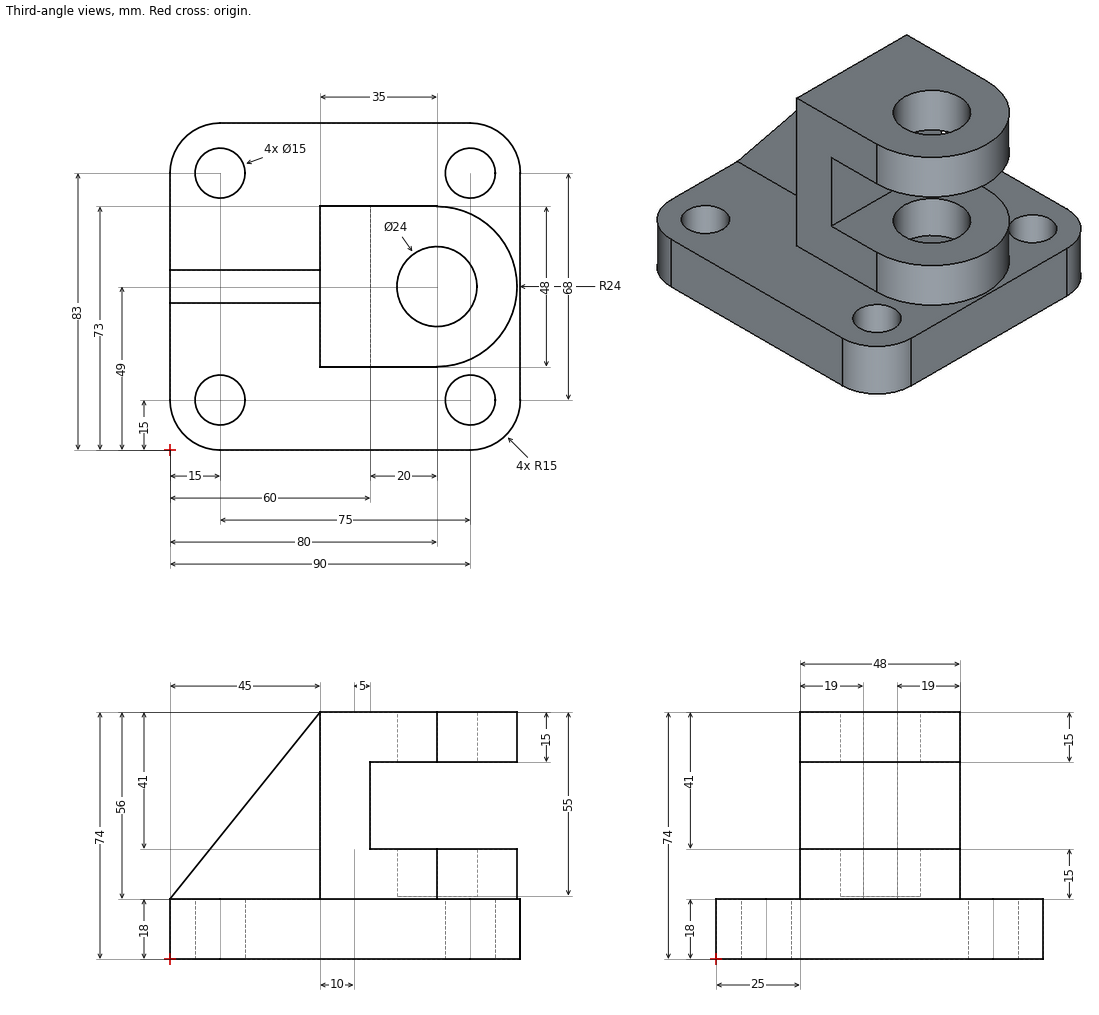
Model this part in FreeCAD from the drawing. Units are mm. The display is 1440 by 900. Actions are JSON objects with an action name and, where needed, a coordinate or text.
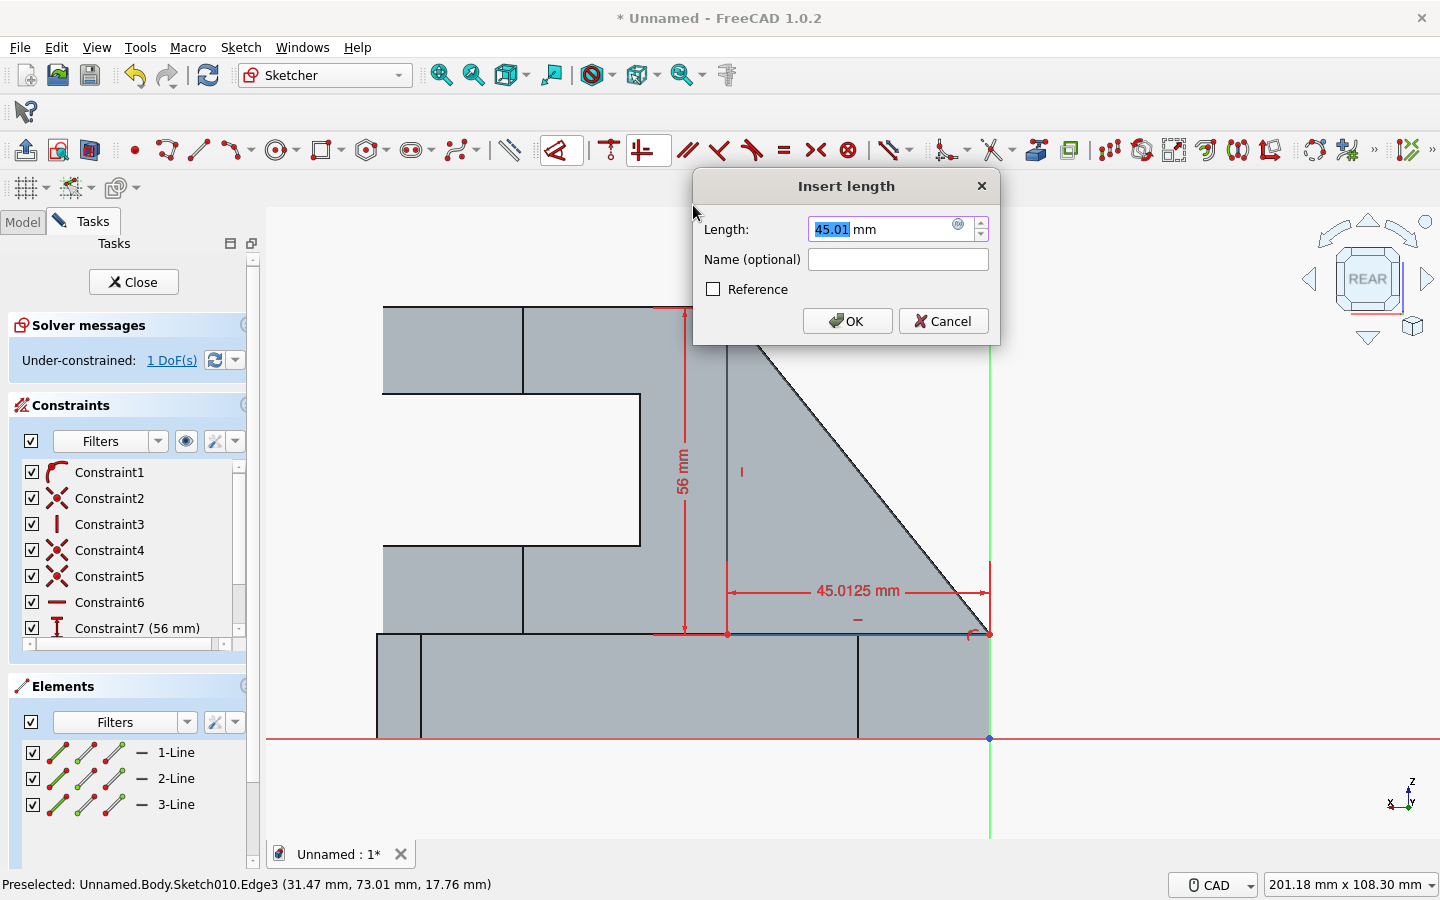
{"action": "type", "text": "45"}
{"action": "key", "text": "Return"}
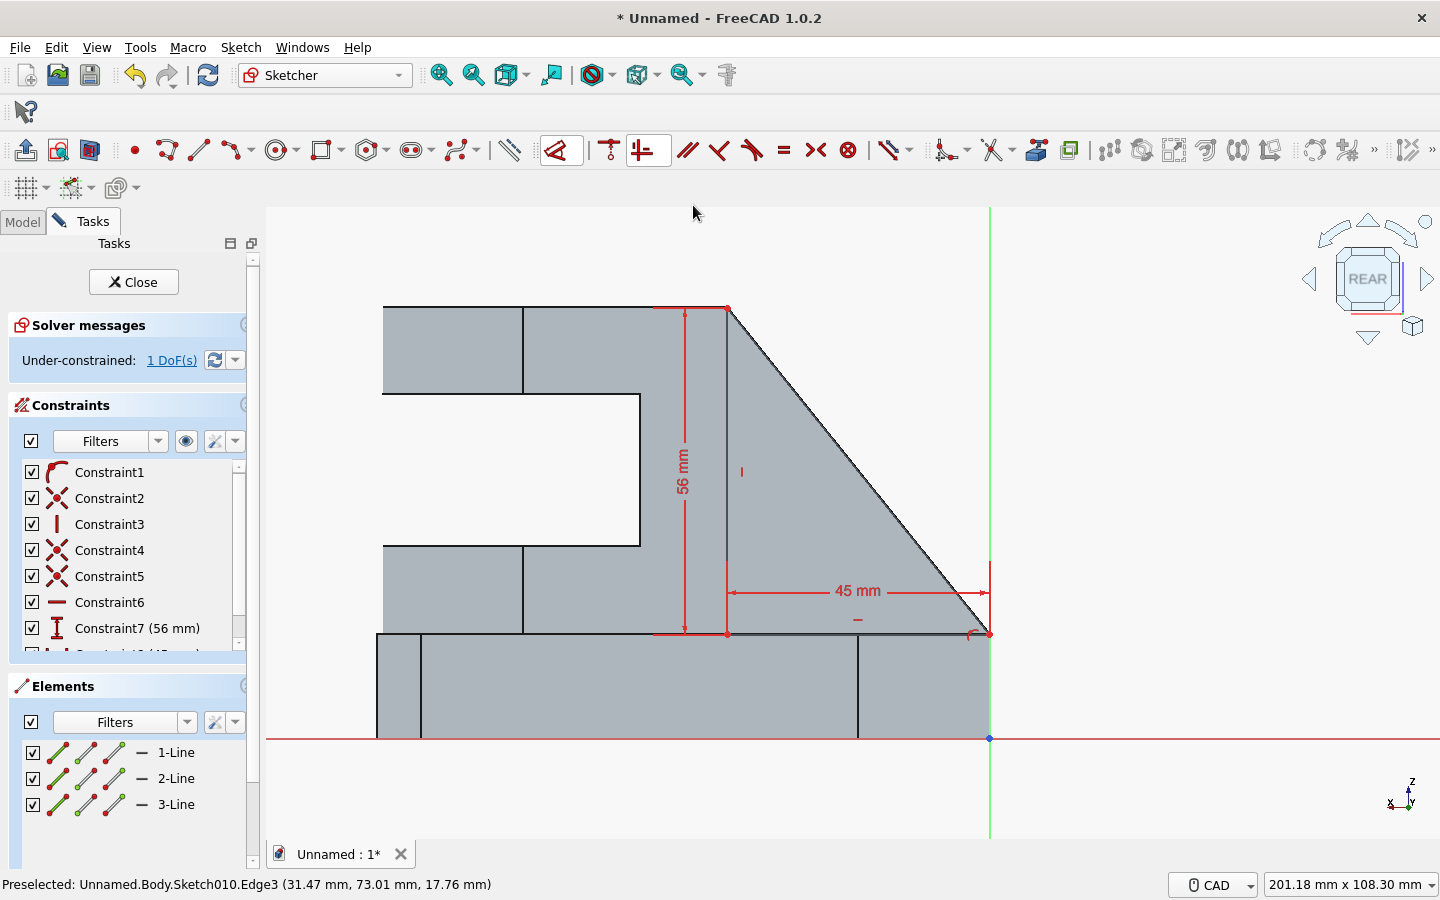
{"action": "left_click", "coordinate": [990, 635]}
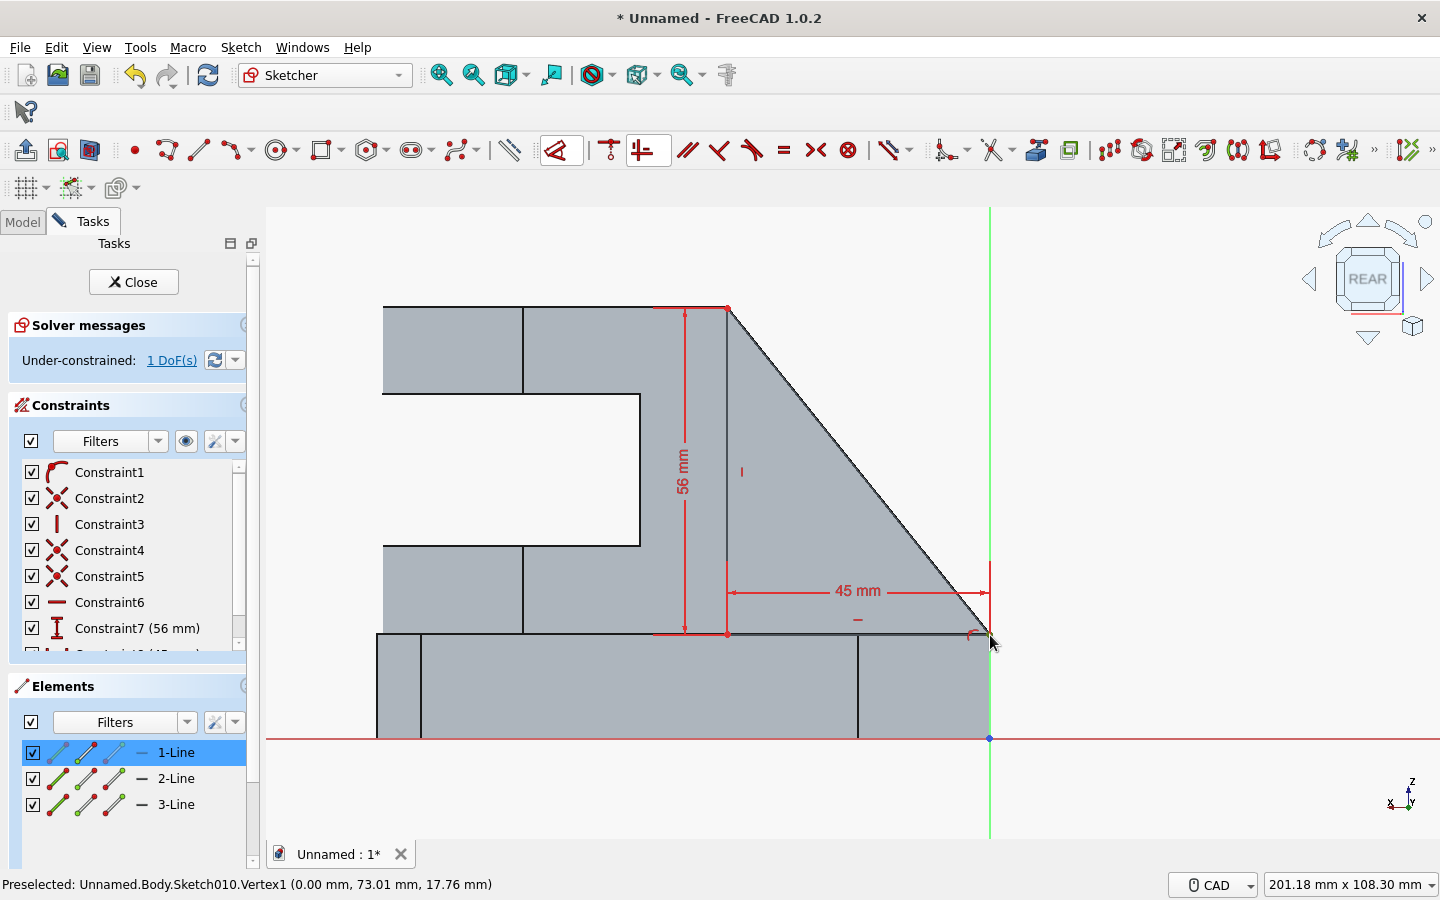
{"action": "left_click", "coordinate": [578, 150]}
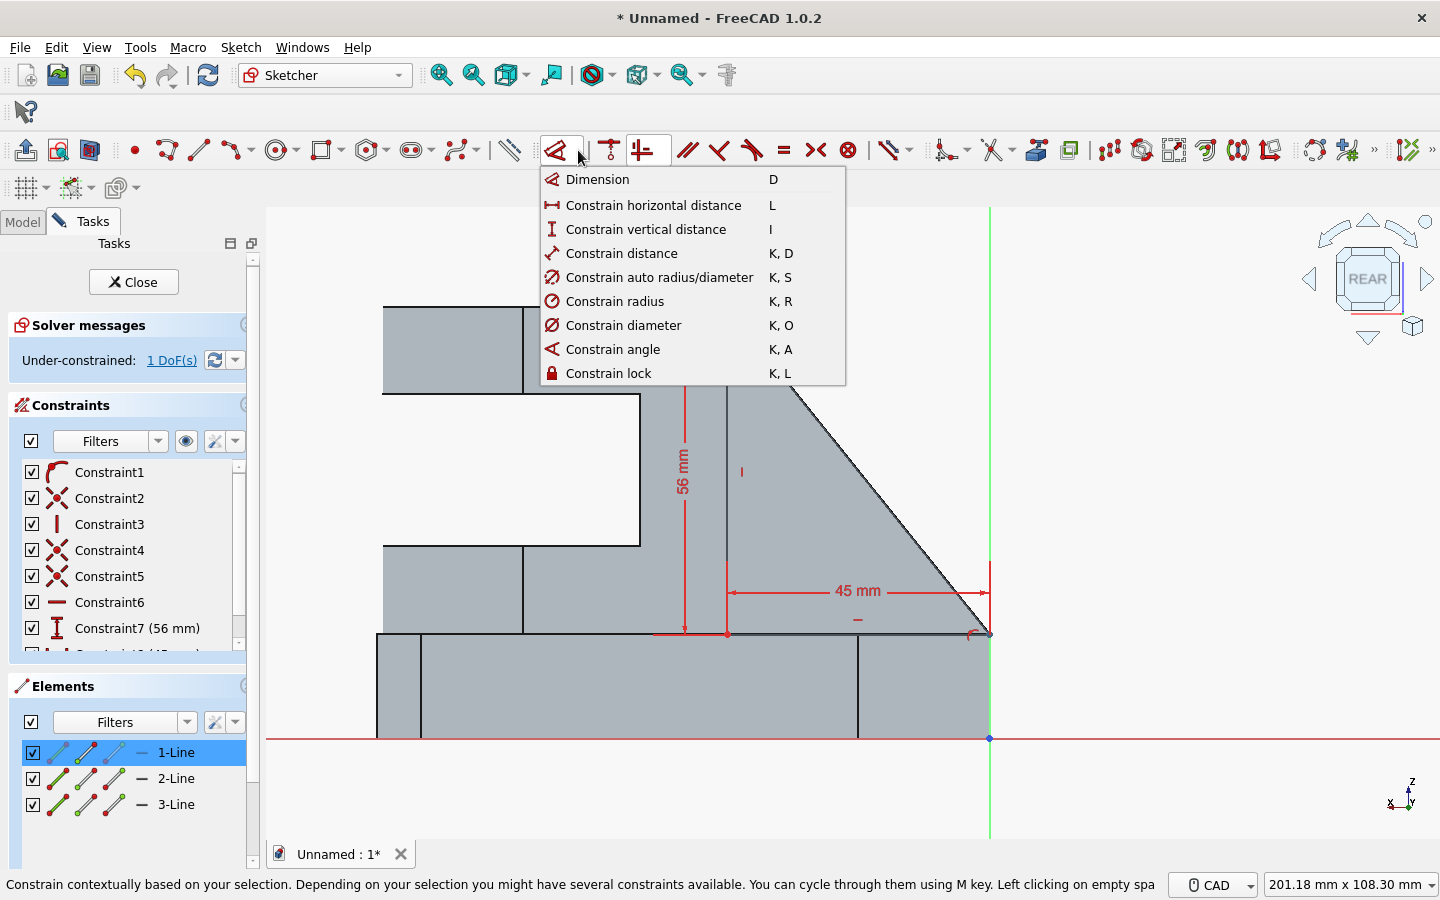
{"action": "left_click", "coordinate": [693, 229]}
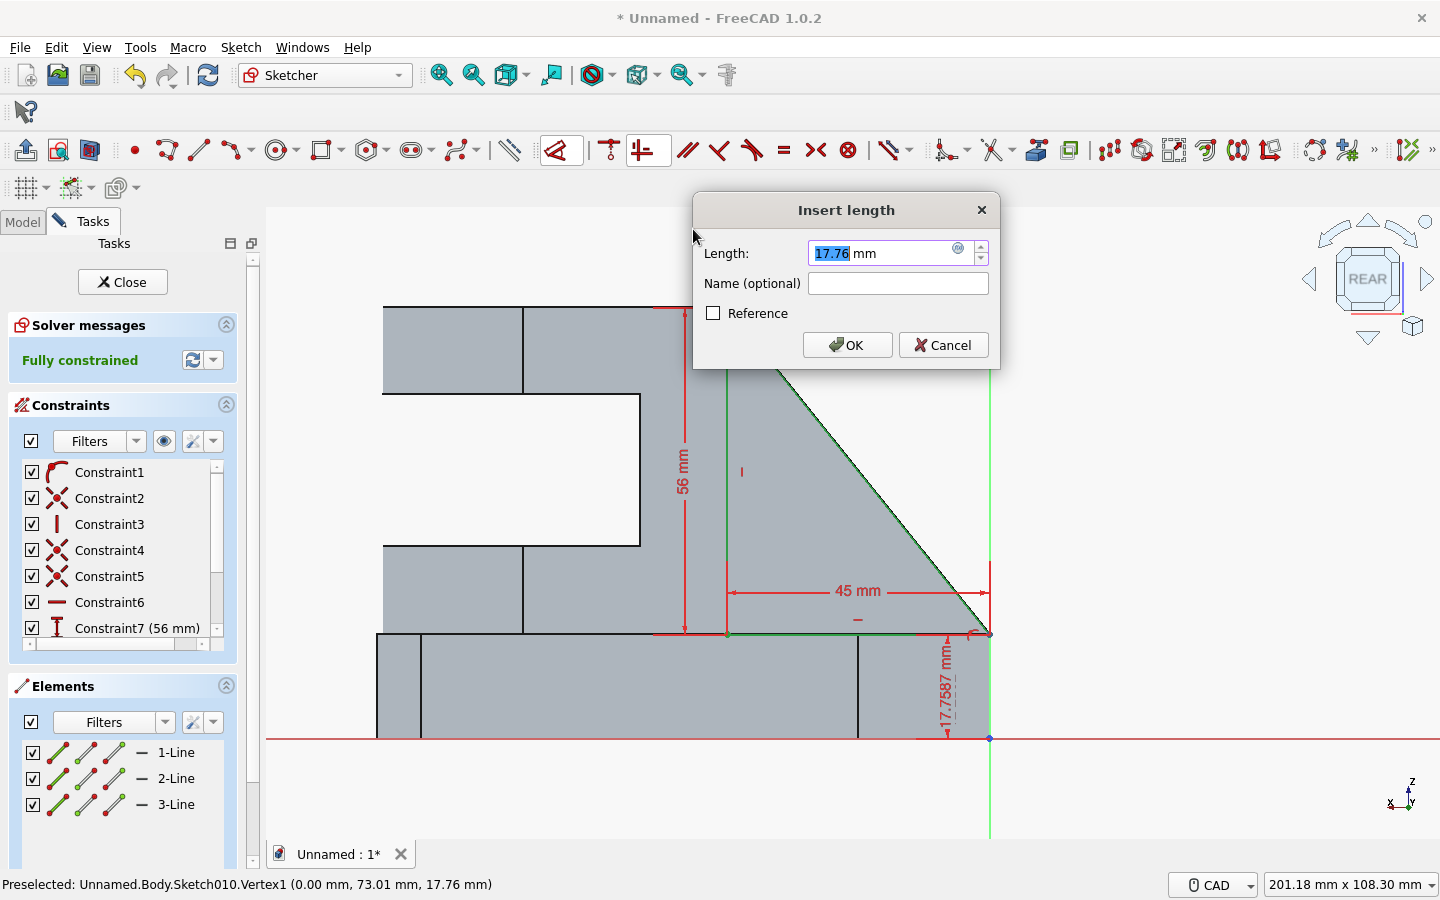
{"action": "type", "text": "18"}
{"action": "key", "text": "Return"}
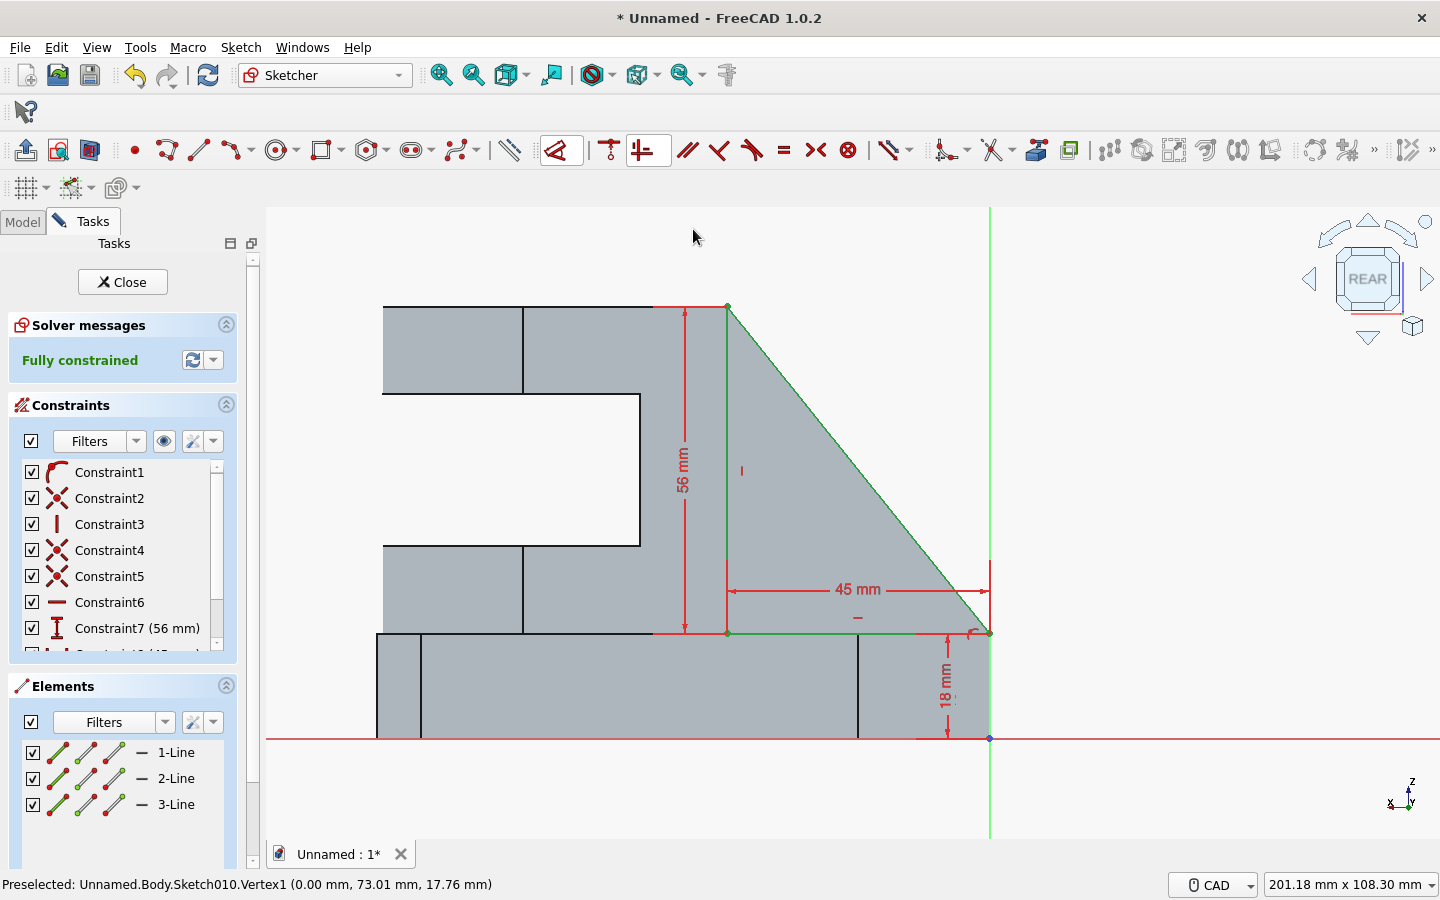
{"action": "left_click", "coordinate": [123, 282]}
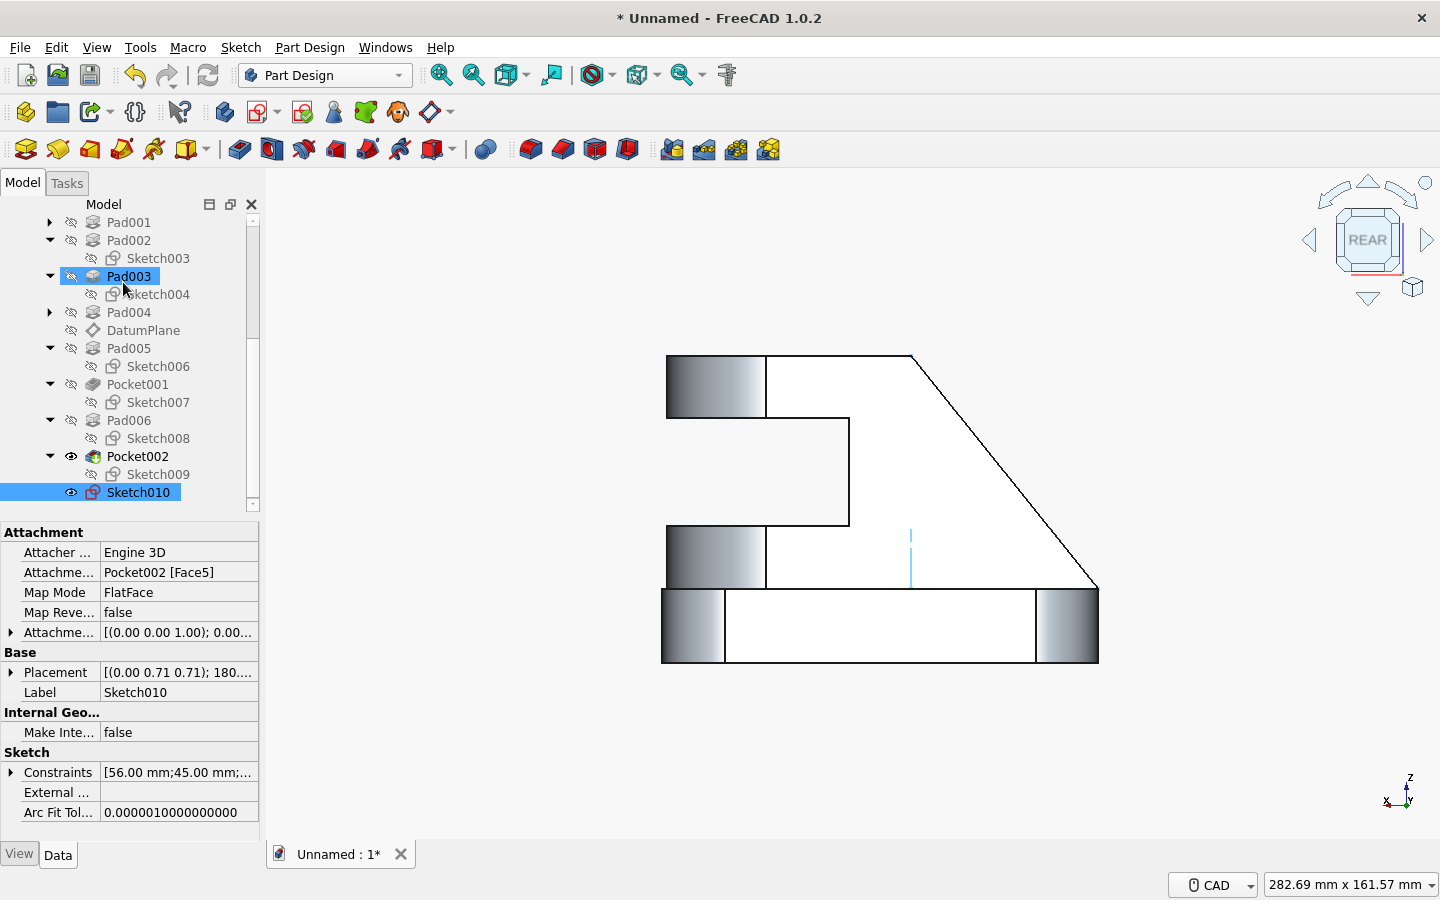
{"action": "left_click", "coordinate": [240, 150]}